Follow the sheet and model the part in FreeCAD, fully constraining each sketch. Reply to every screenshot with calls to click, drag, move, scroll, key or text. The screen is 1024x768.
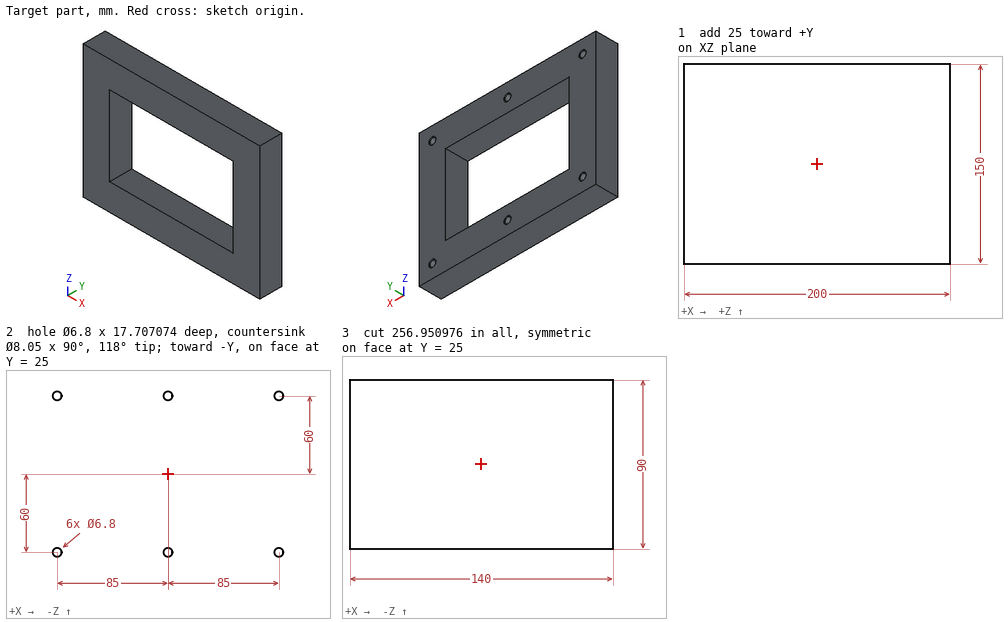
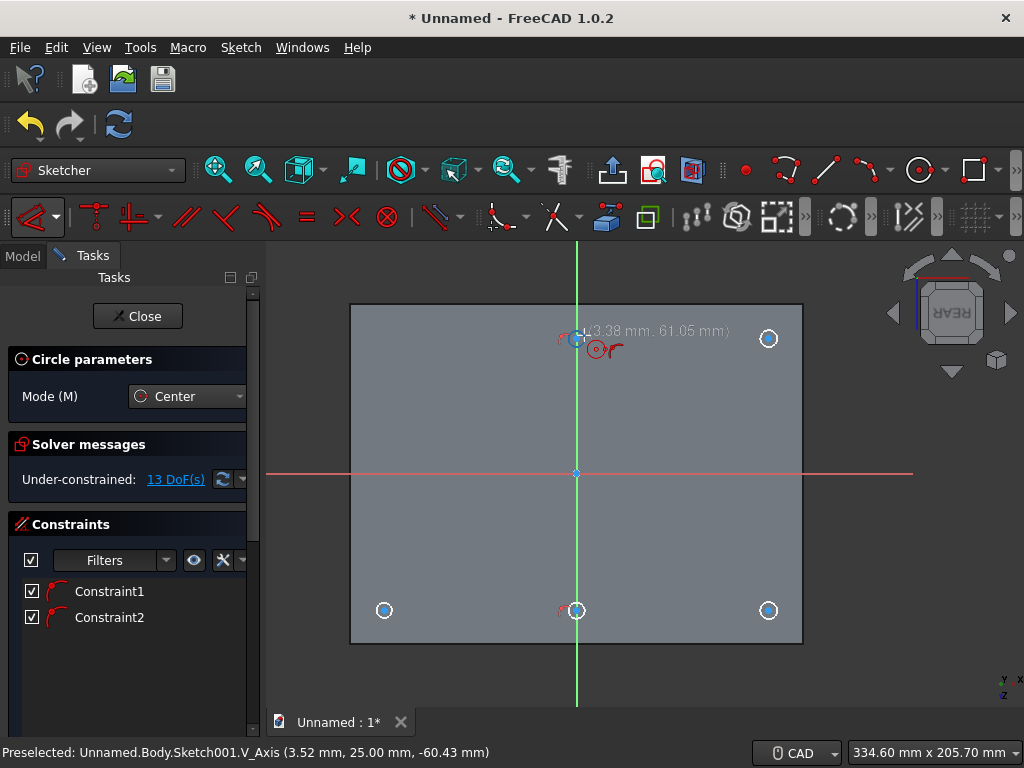
scroll(384, 338, up, 6)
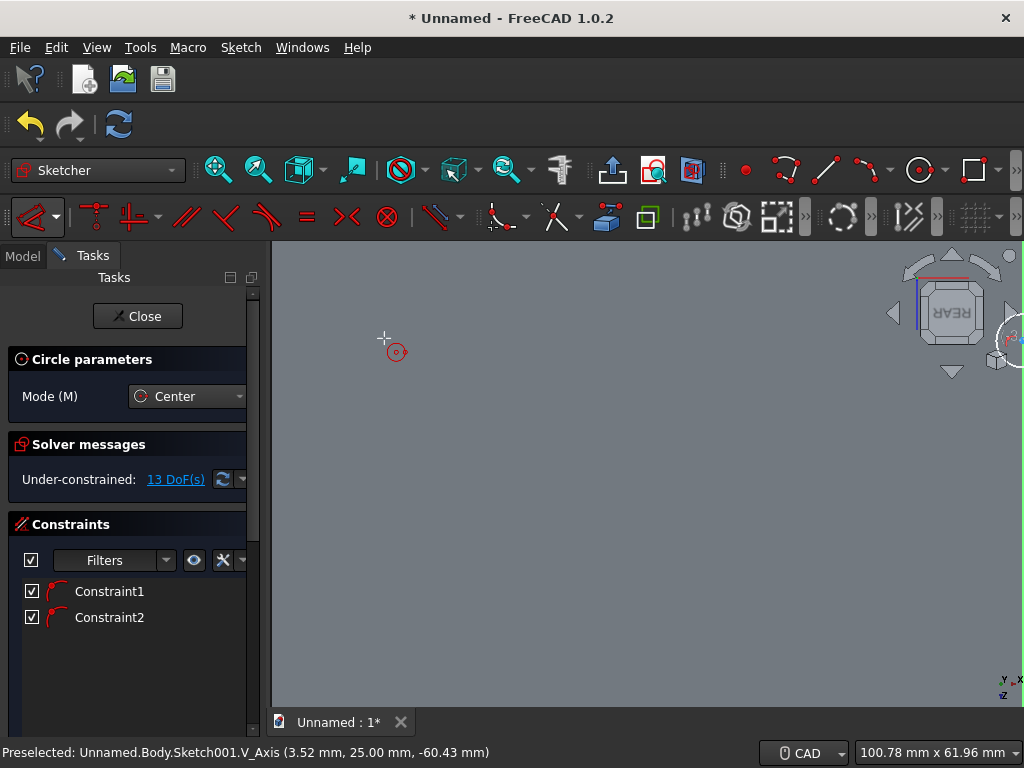
scroll(384, 338, down, 6)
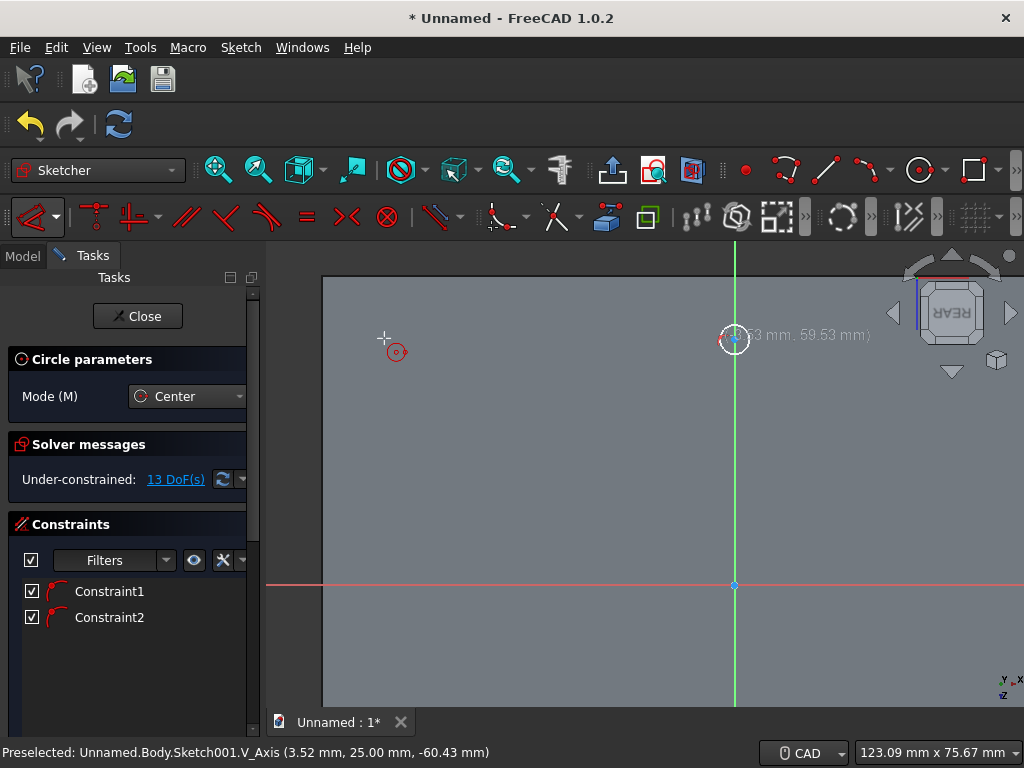
click(384, 338)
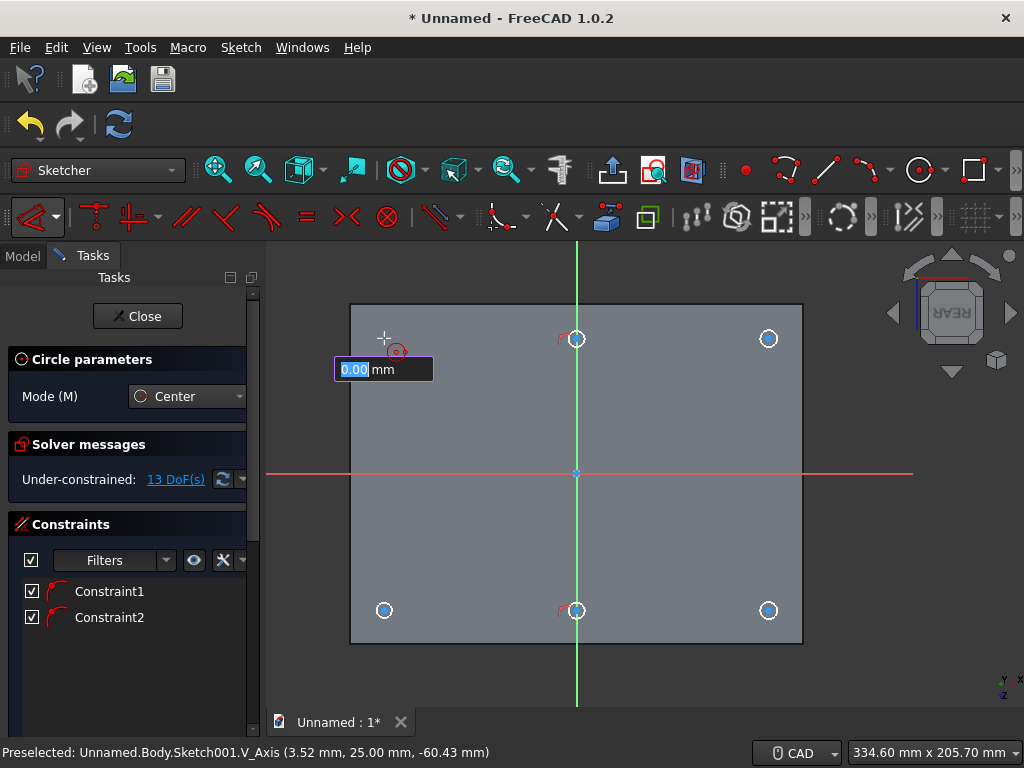
scroll(389, 332, up, 4)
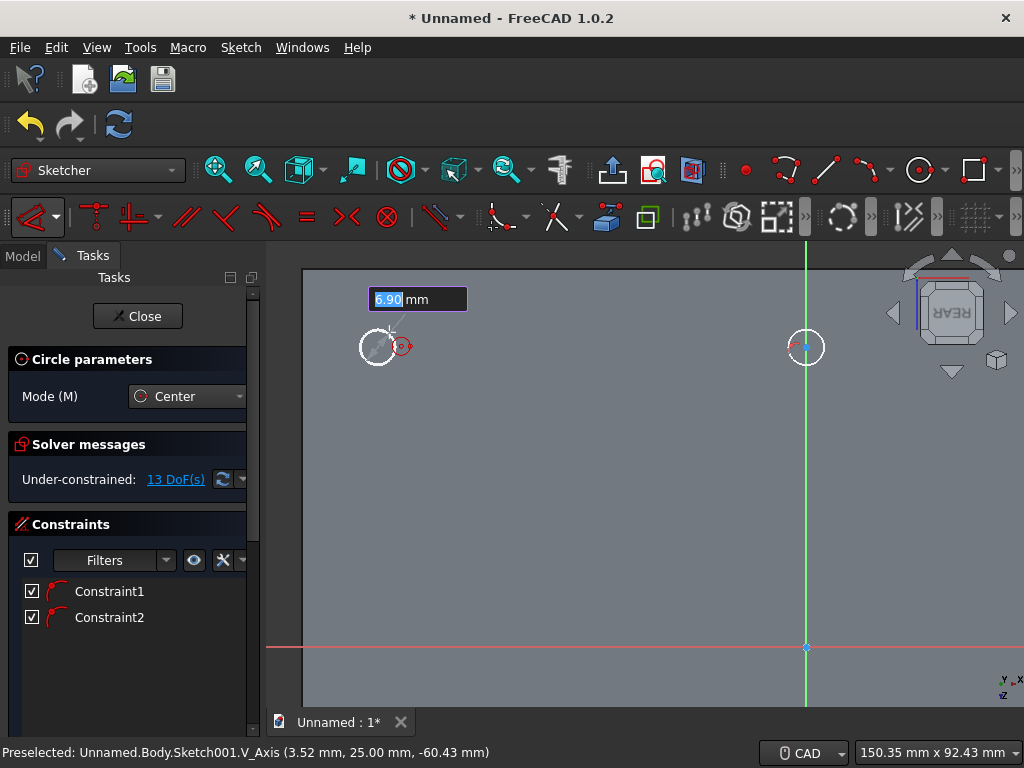
click(390, 333)
key(Escape)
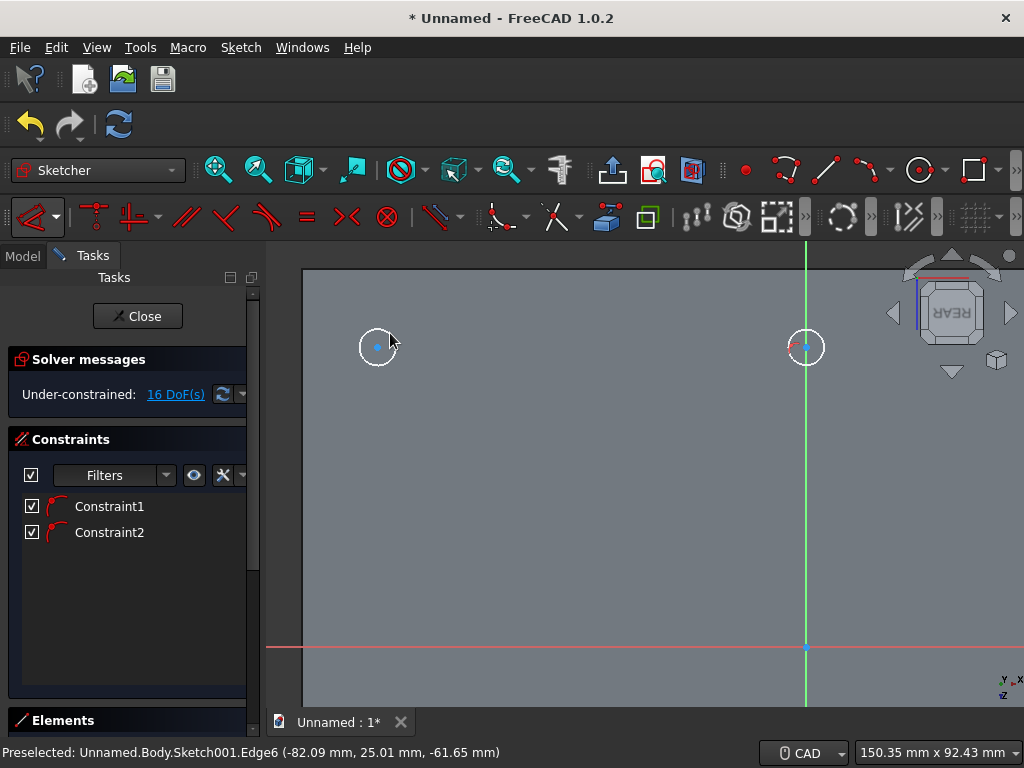
scroll(389, 332, down, 4)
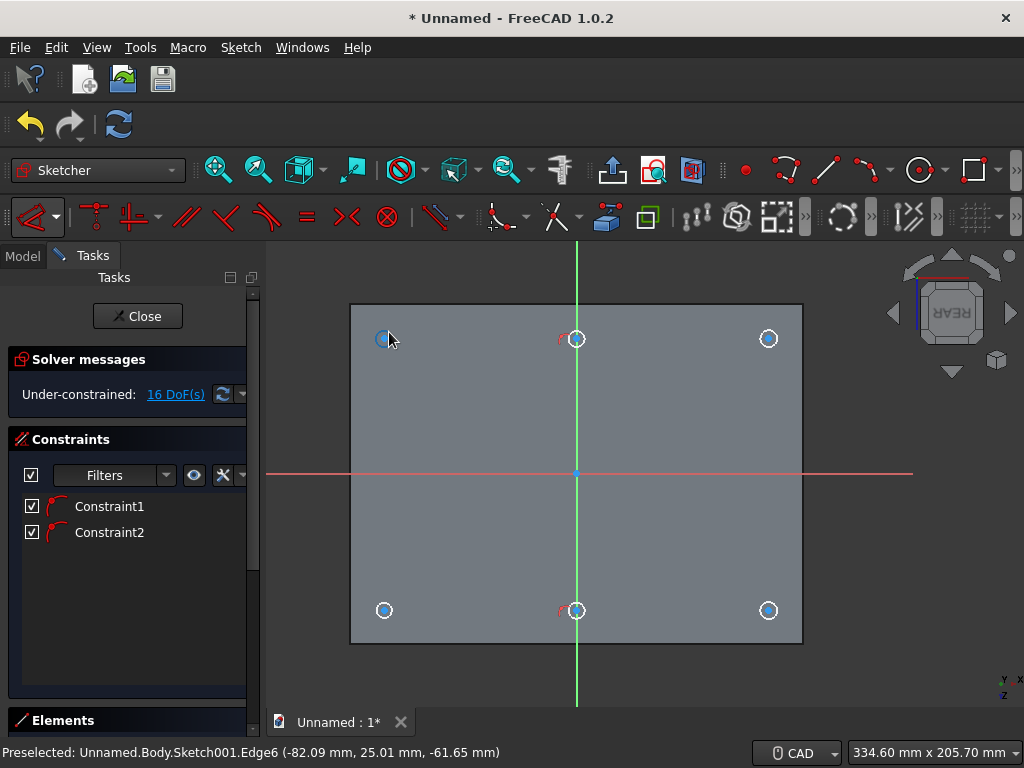
scroll(390, 605, up, 4)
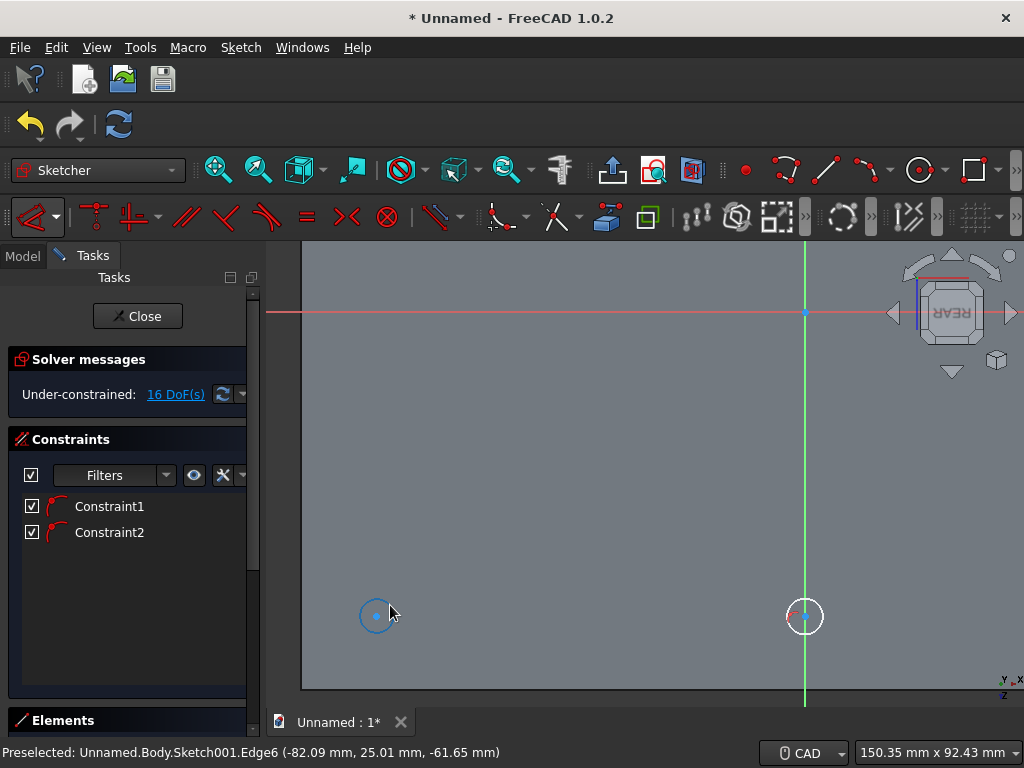
click(389, 604)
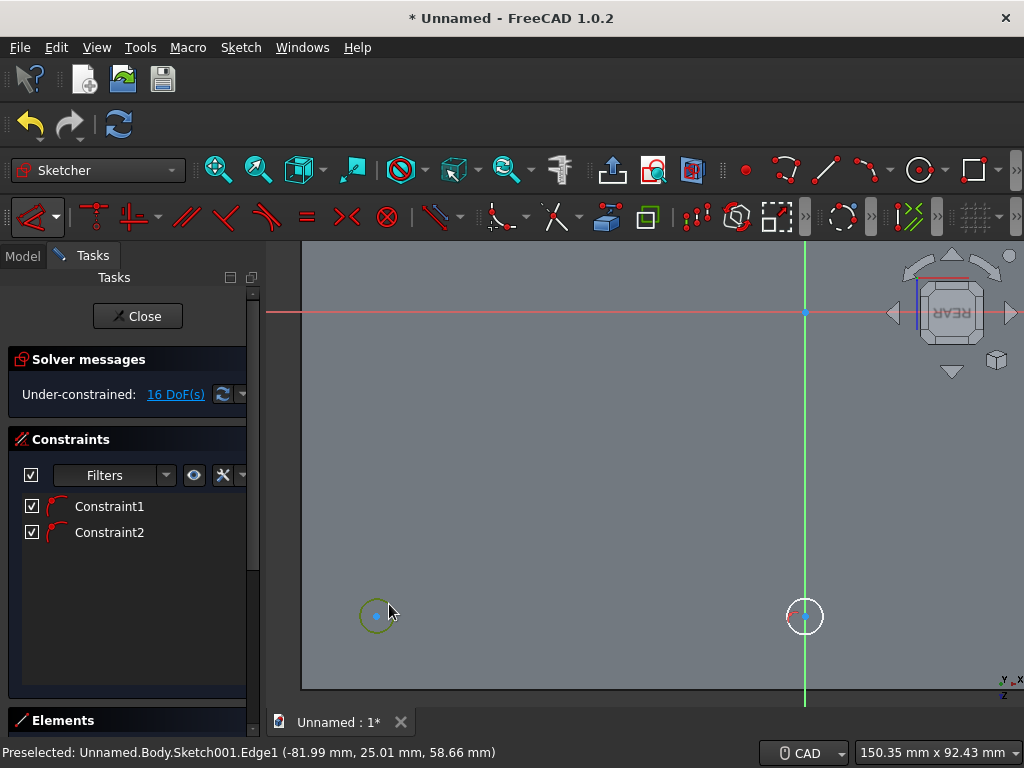
click(818, 604)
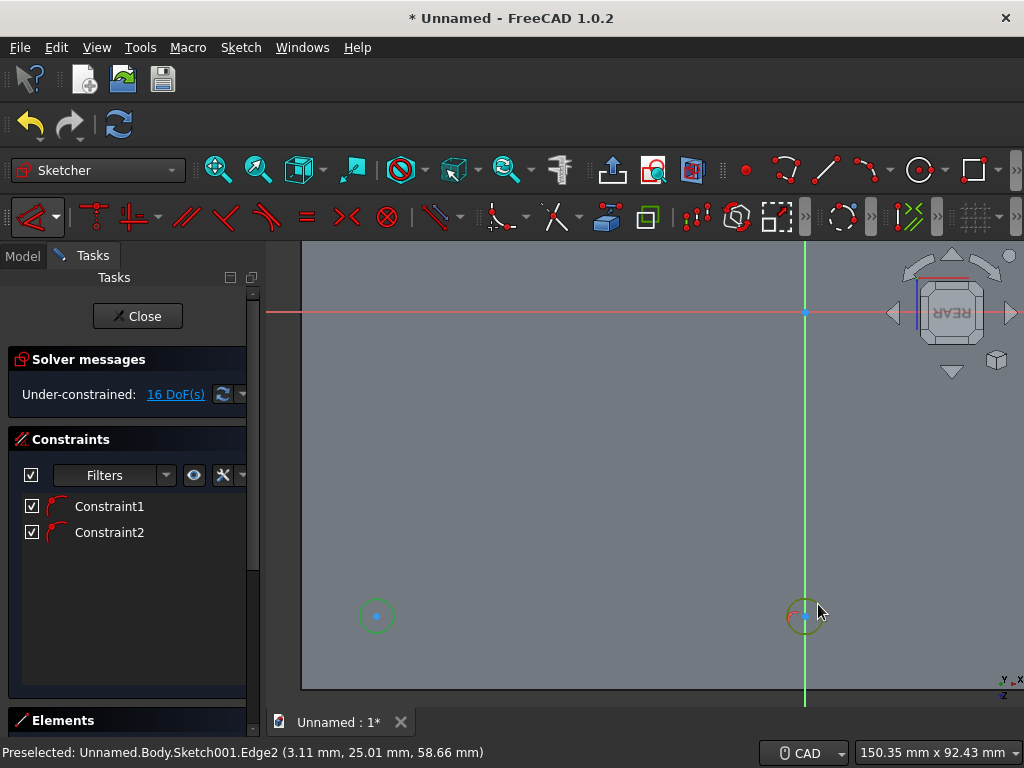
scroll(390, 606, down, 4)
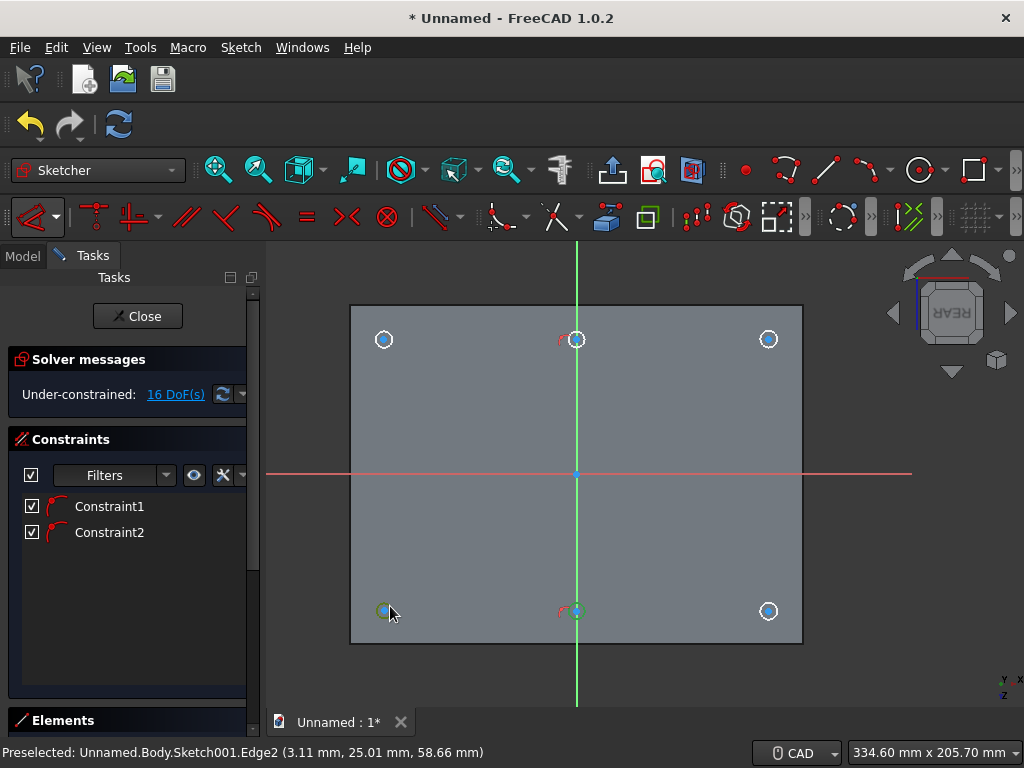
scroll(775, 605, up, 3)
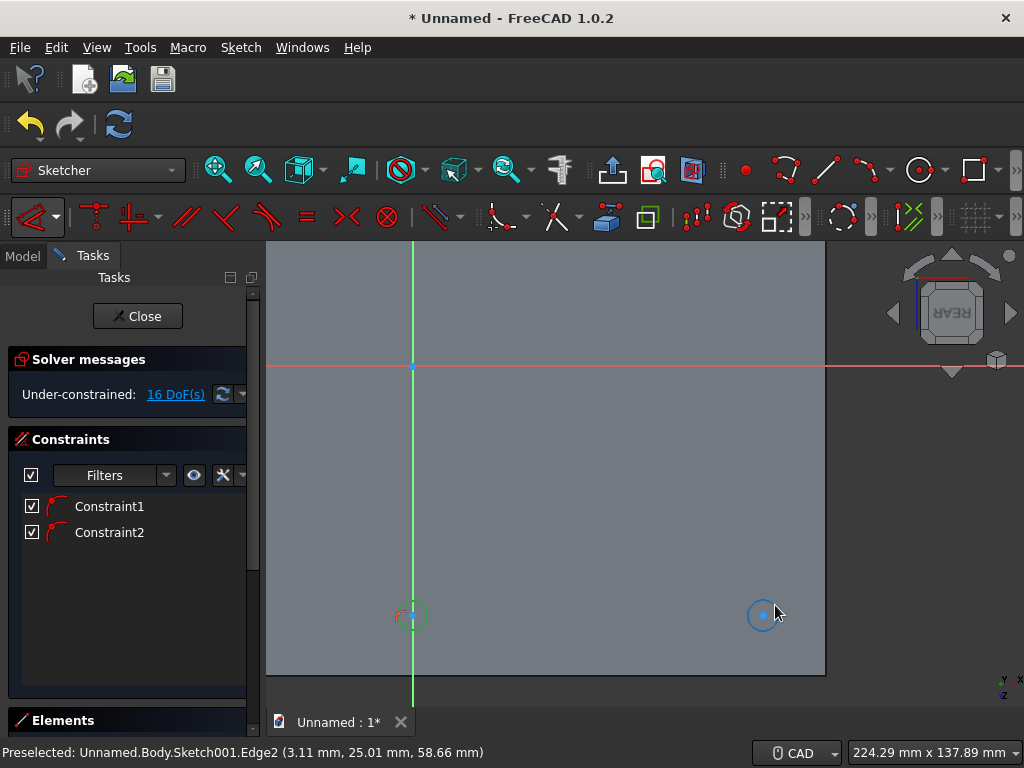
click(774, 605)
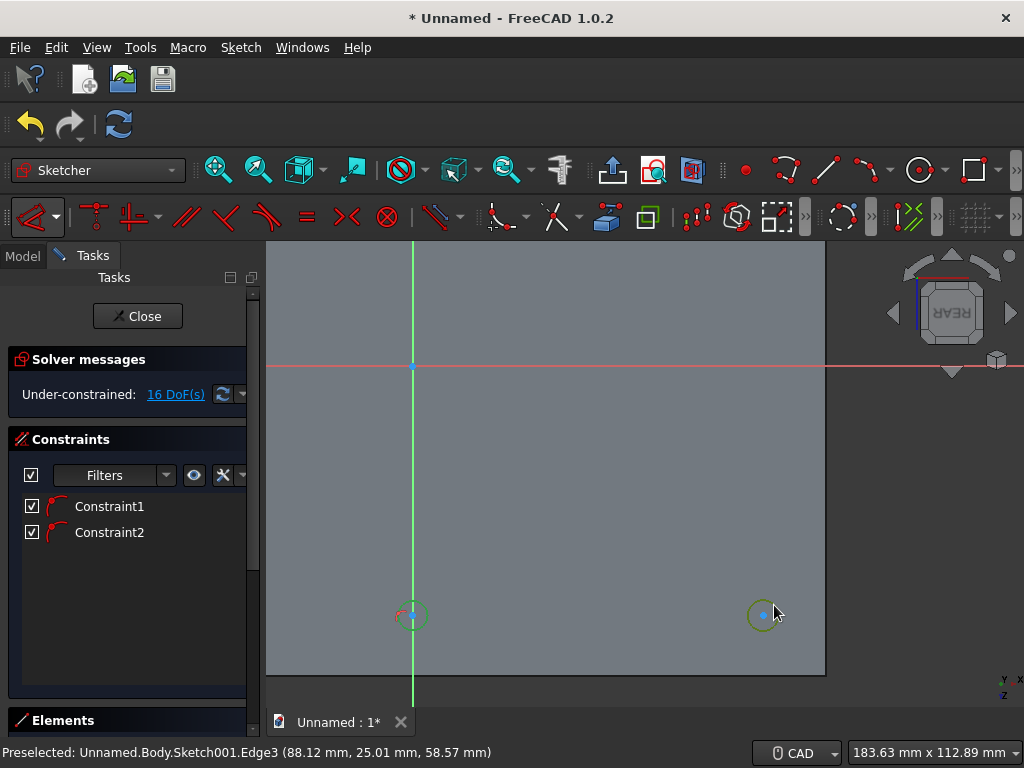
scroll(776, 605, down, 3)